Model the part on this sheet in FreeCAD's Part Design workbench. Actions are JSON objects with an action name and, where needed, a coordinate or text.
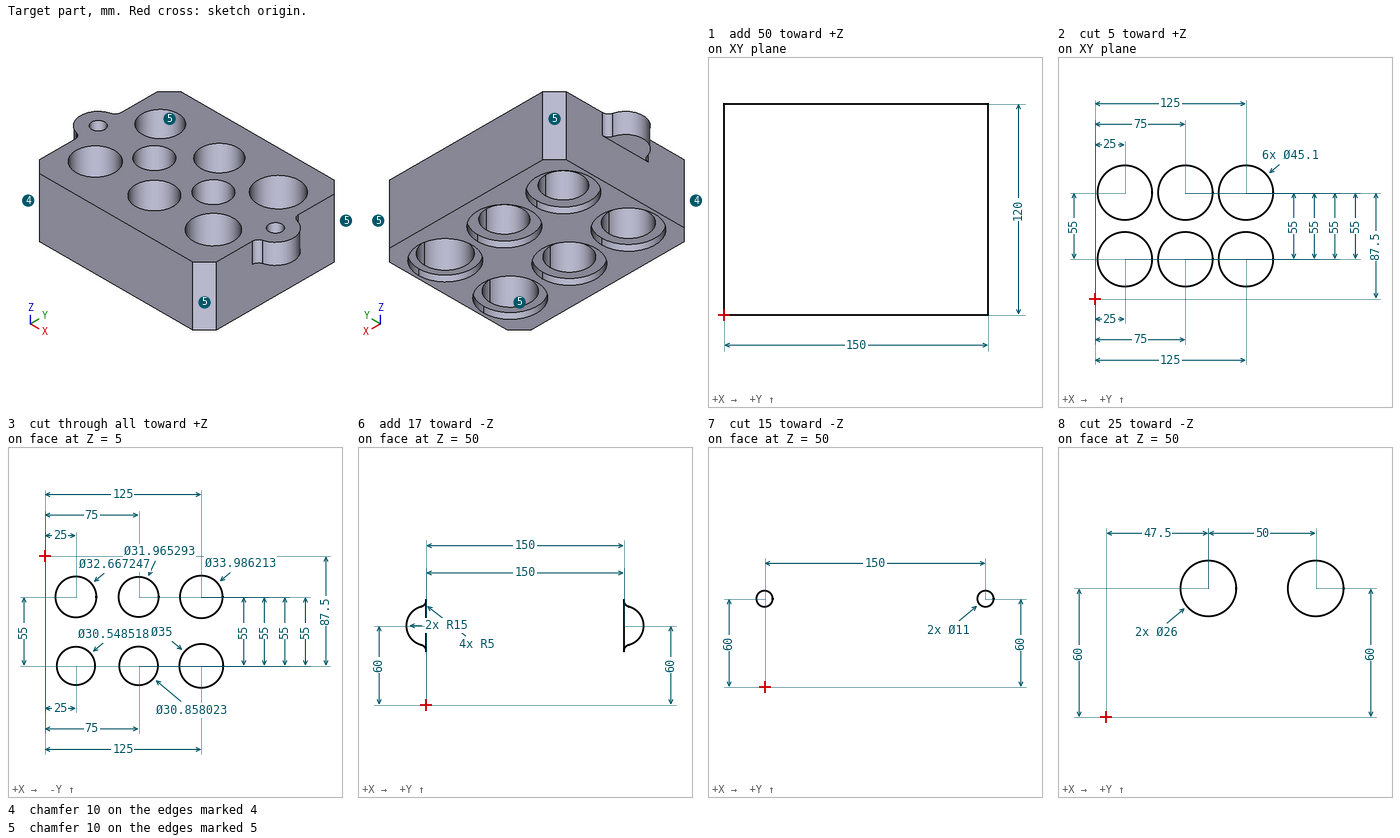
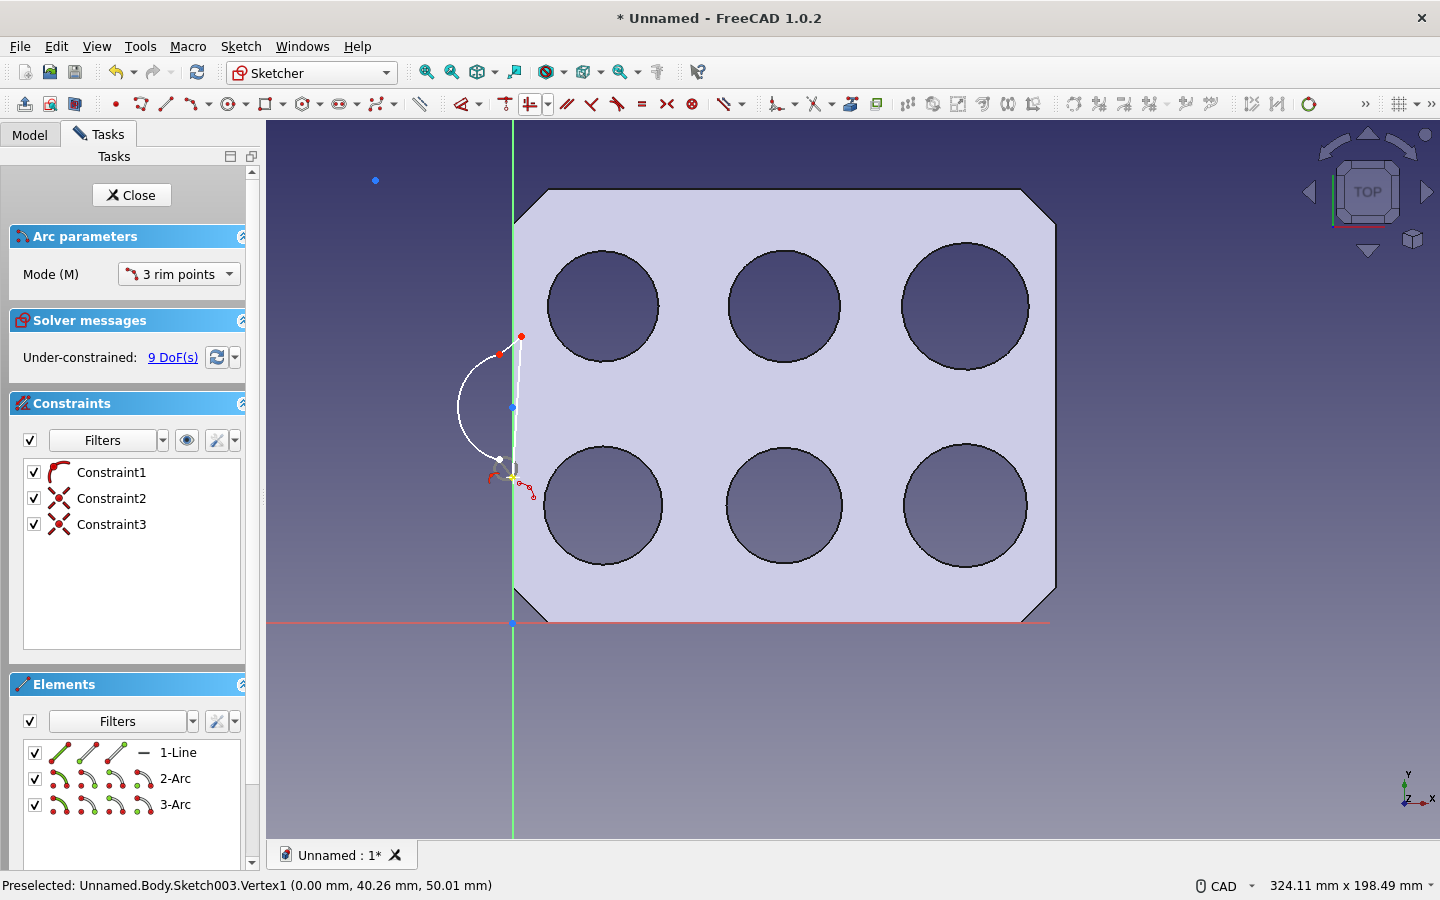
{"action": "scroll", "coordinate": [509, 465], "scroll_direction": "up", "scroll_amount": 8}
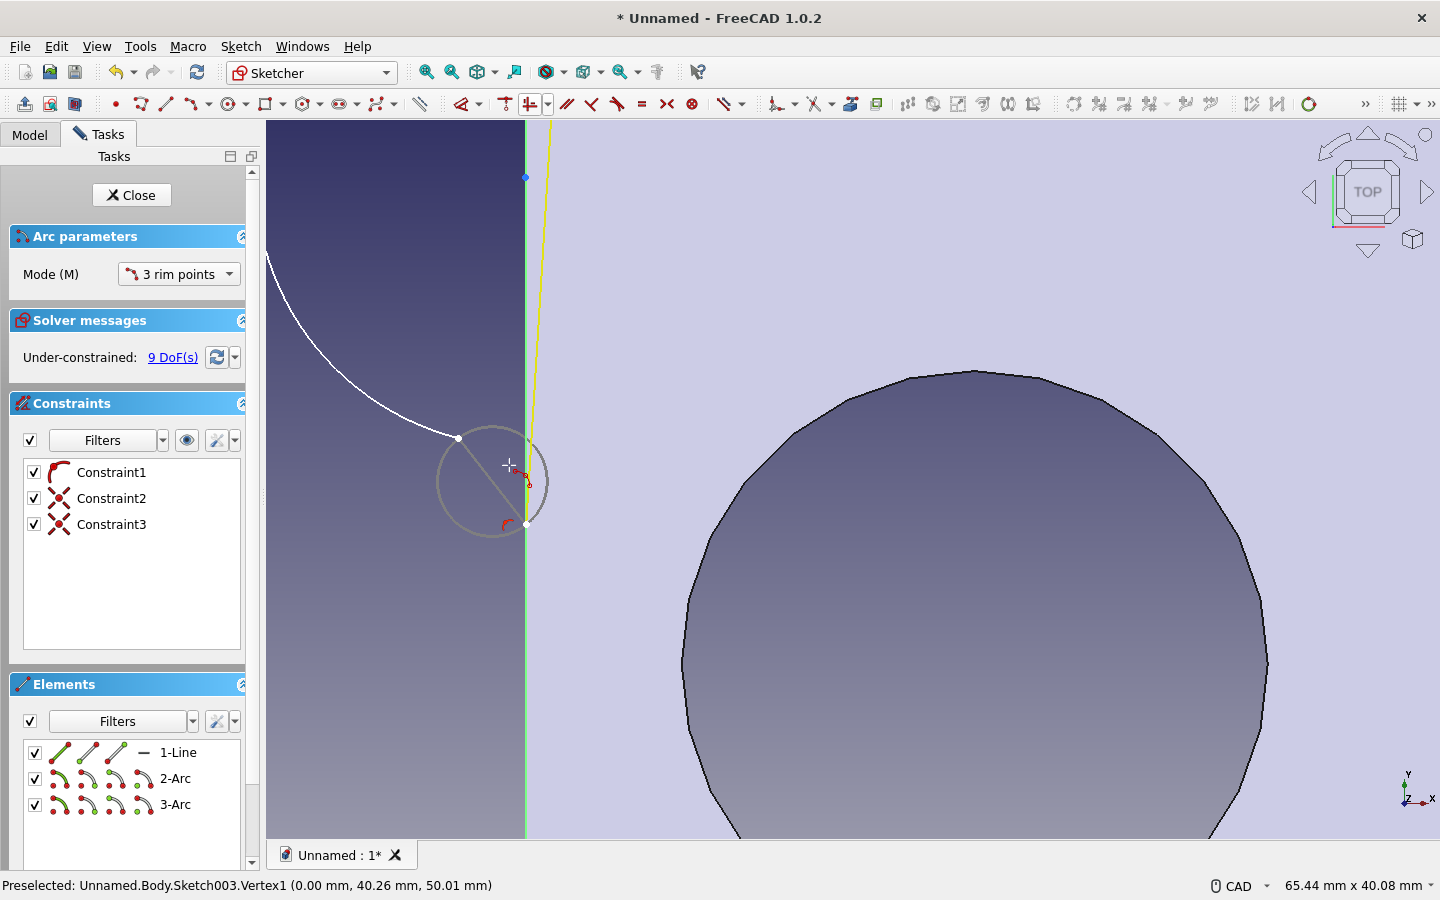
{"action": "left_click", "coordinate": [507, 463]}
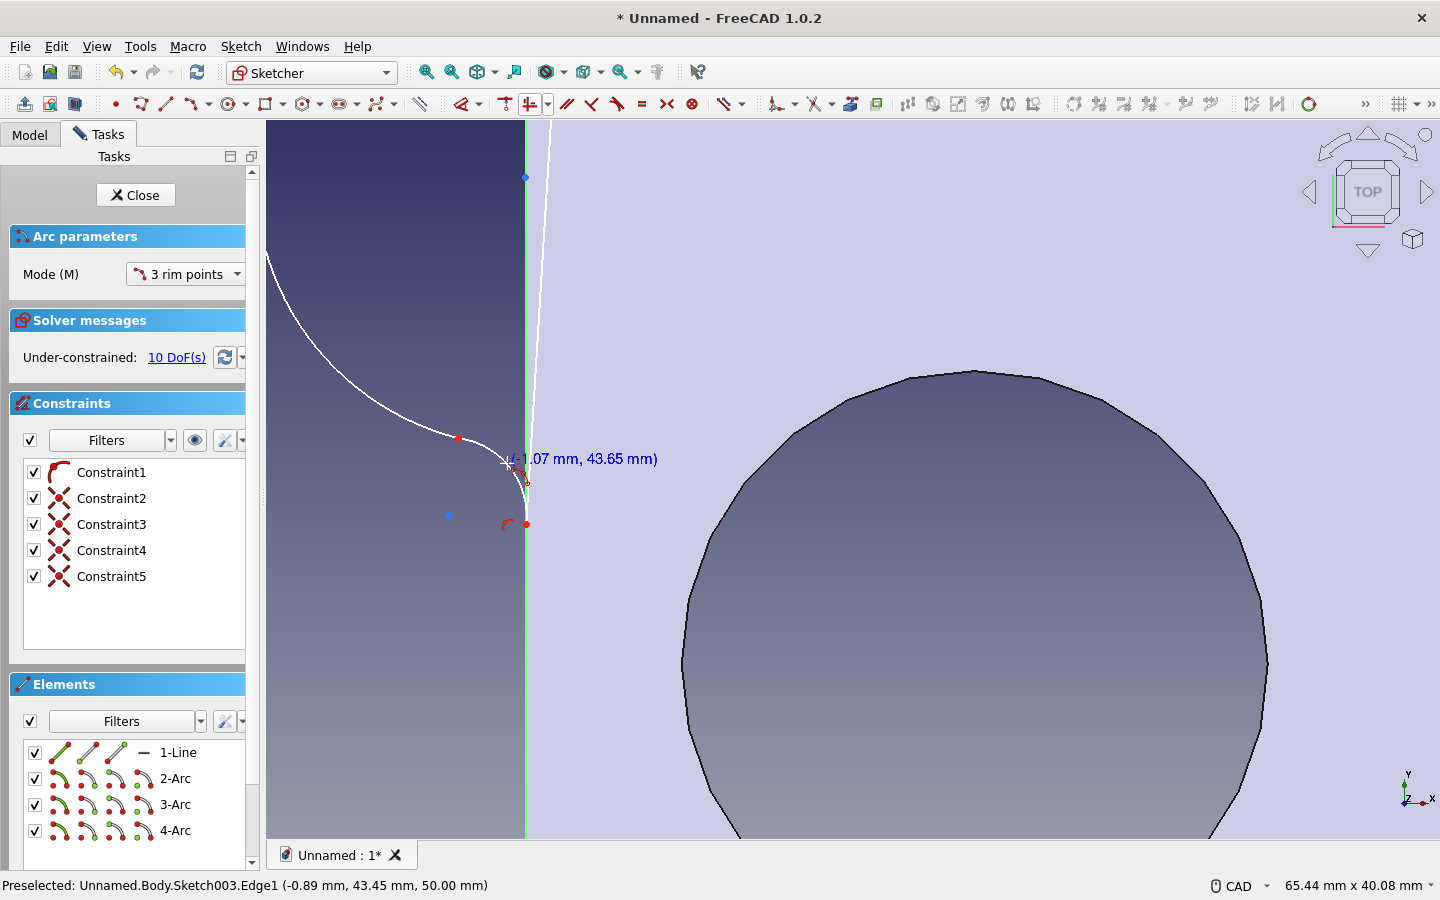
{"action": "left_click", "coordinate": [166, 104]}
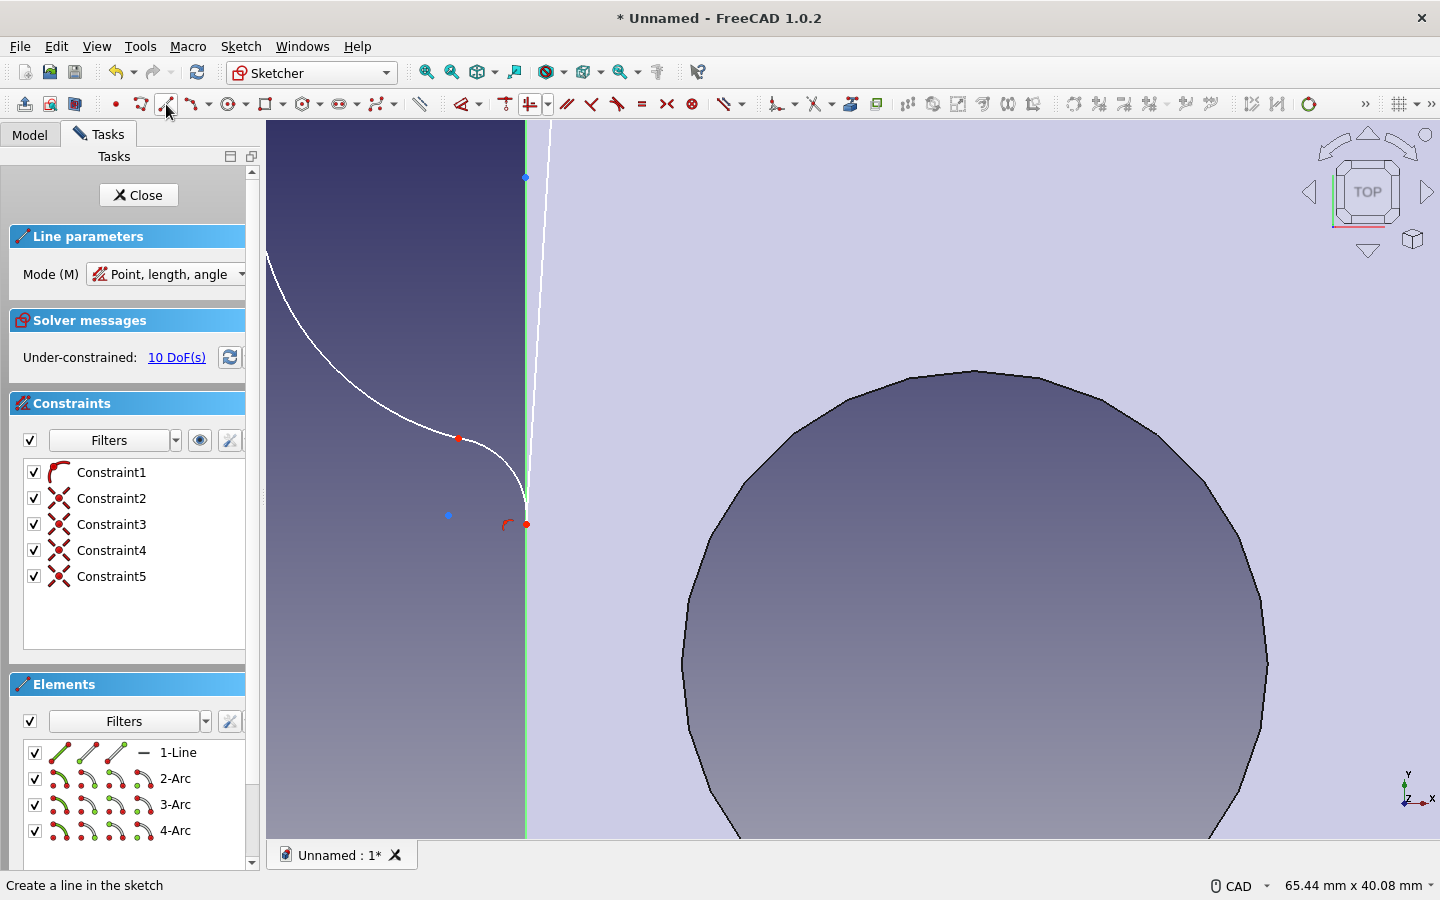
{"action": "scroll", "coordinate": [509, 465], "scroll_direction": "down", "scroll_amount": 8}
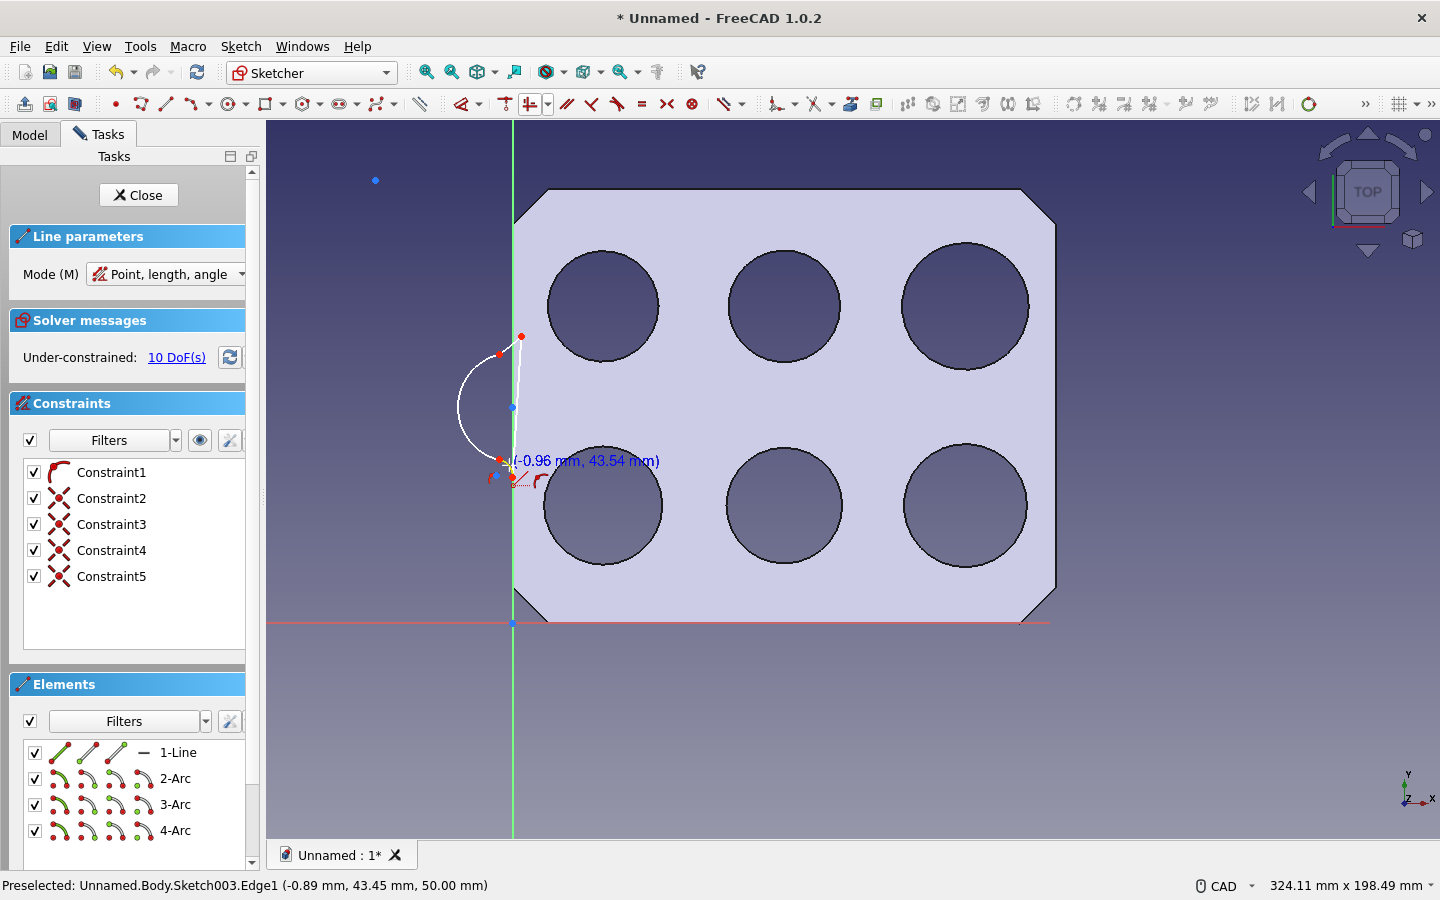
{"action": "left_click", "coordinate": [1056, 336]}
{"action": "left_click", "coordinate": [1056, 476]}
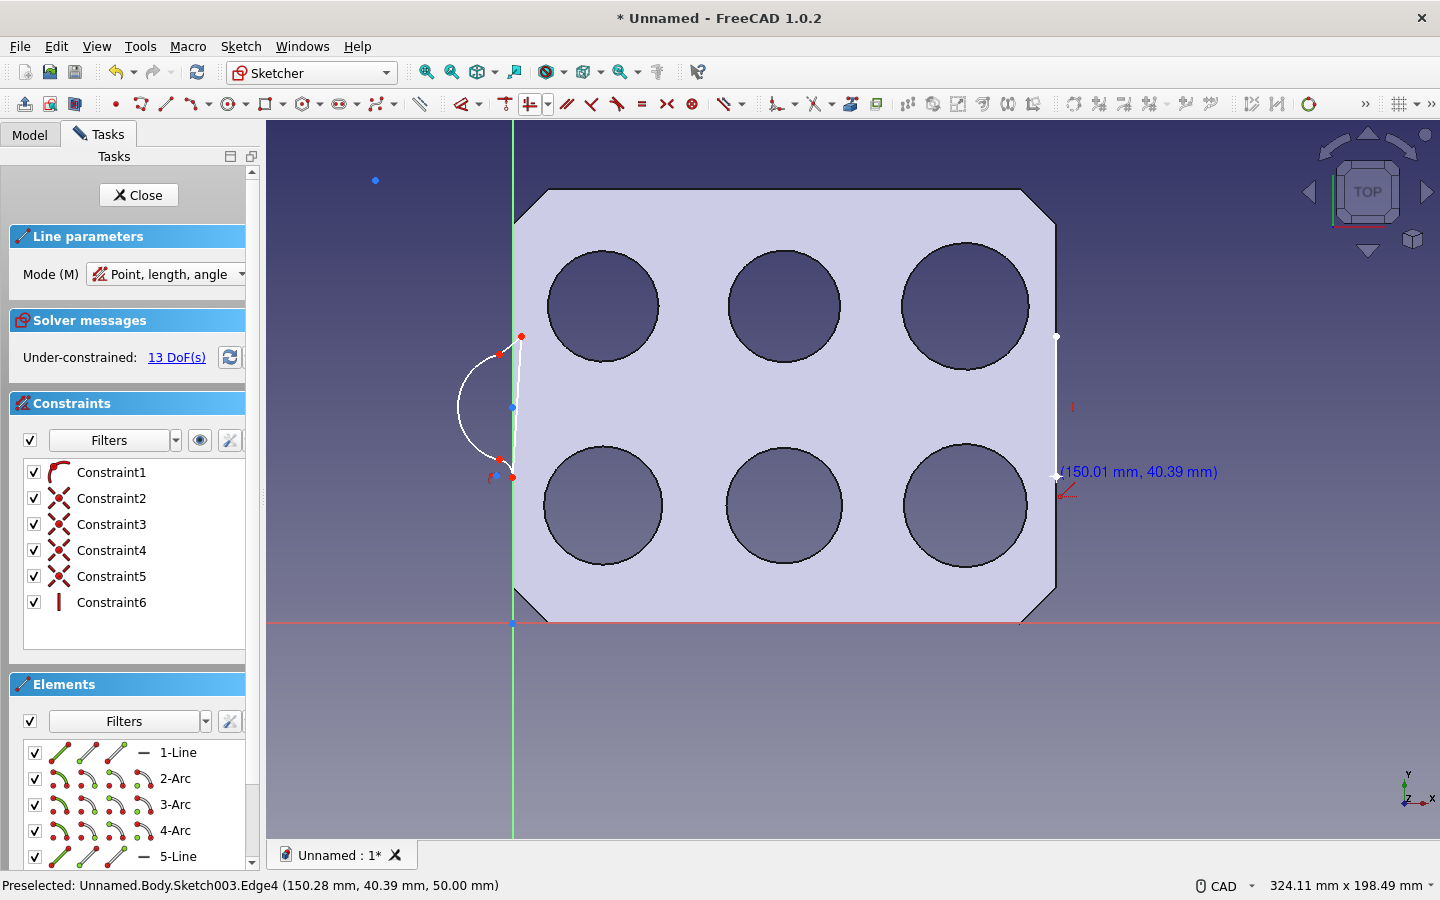
{"action": "left_click", "coordinate": [190, 104]}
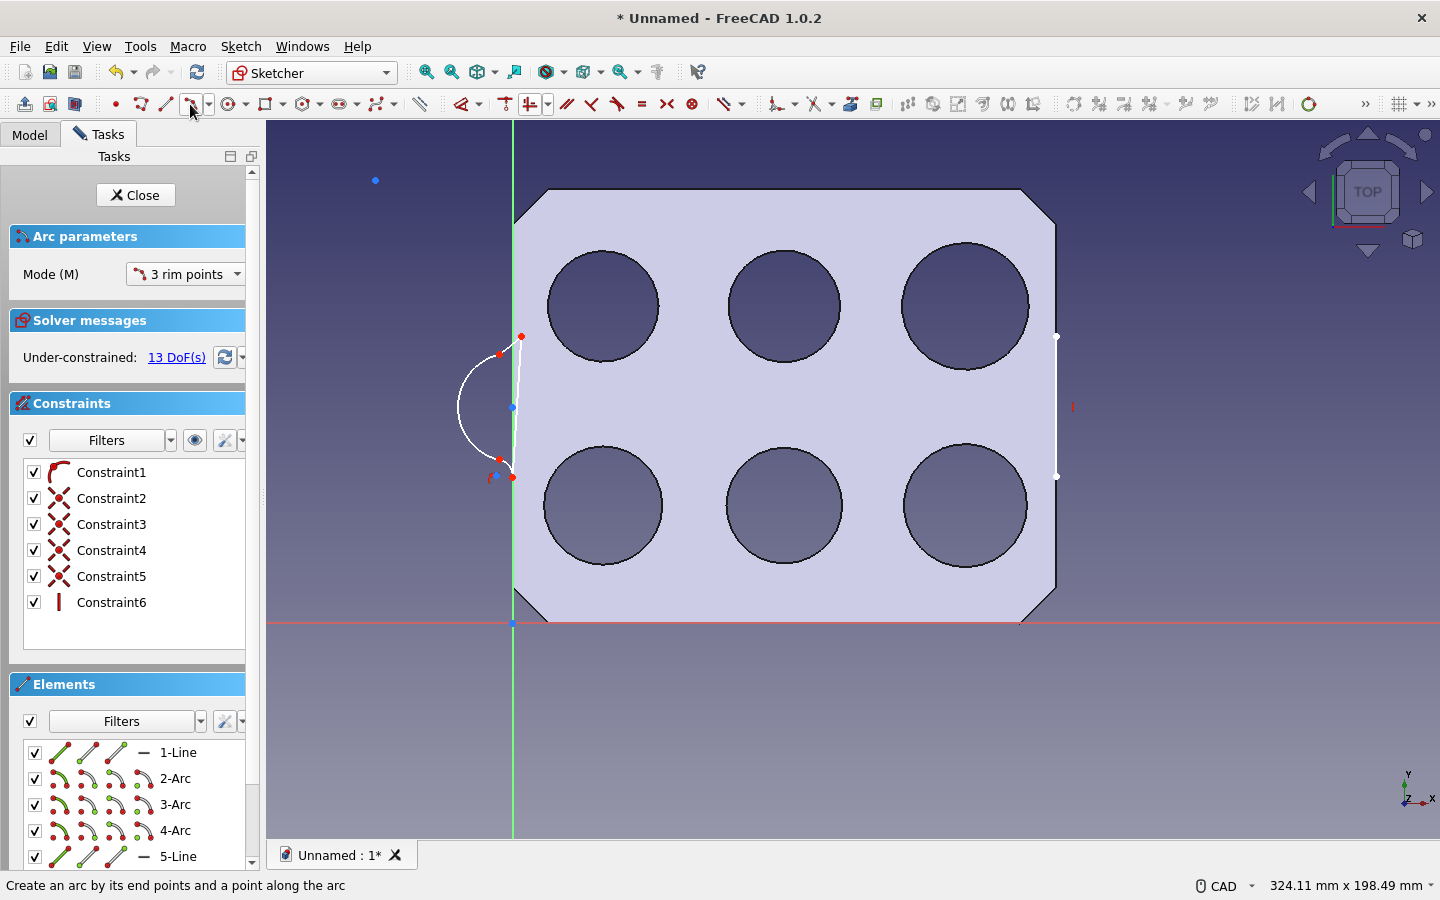
{"action": "left_click", "coordinate": [1056, 477]}
{"action": "left_click", "coordinate": [1070, 459]}